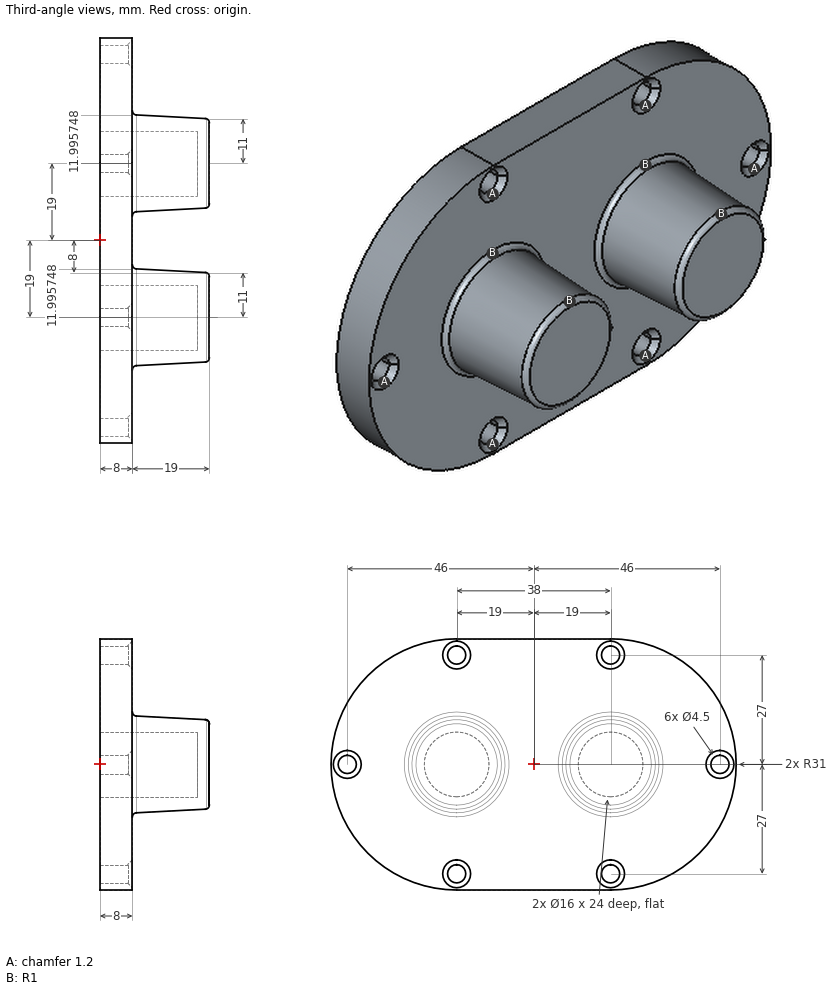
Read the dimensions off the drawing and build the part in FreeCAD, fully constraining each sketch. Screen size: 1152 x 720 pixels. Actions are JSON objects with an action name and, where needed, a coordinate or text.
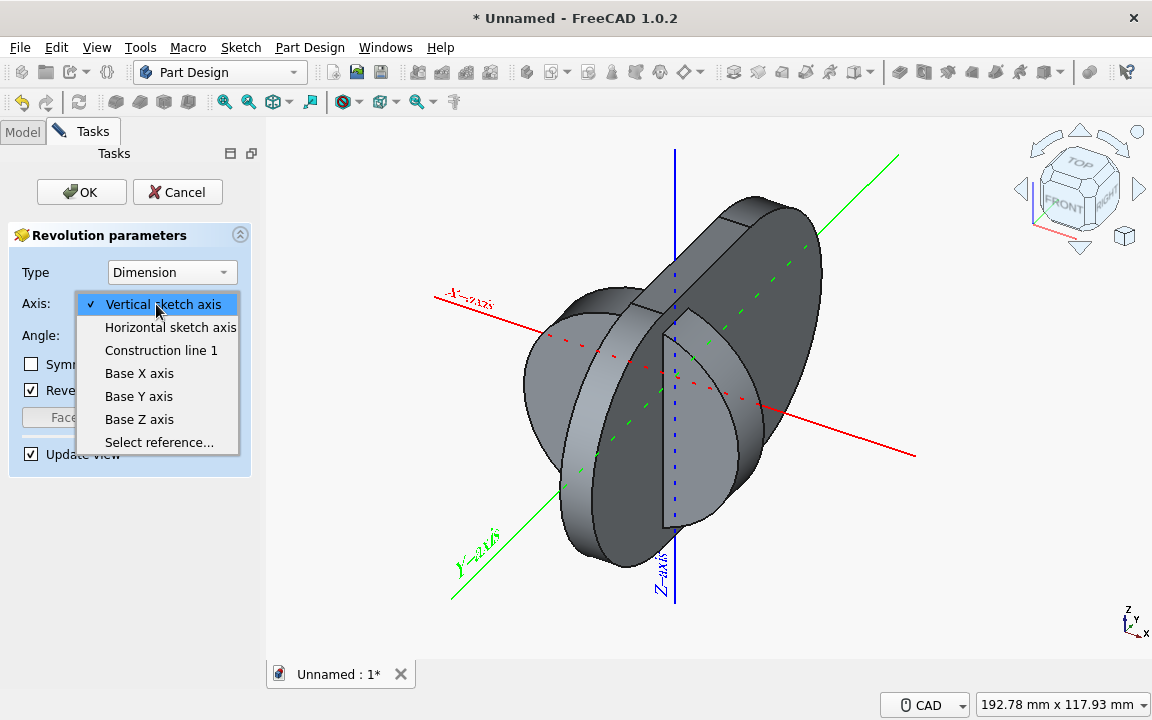
{"action": "left_click", "coordinate": [156, 350]}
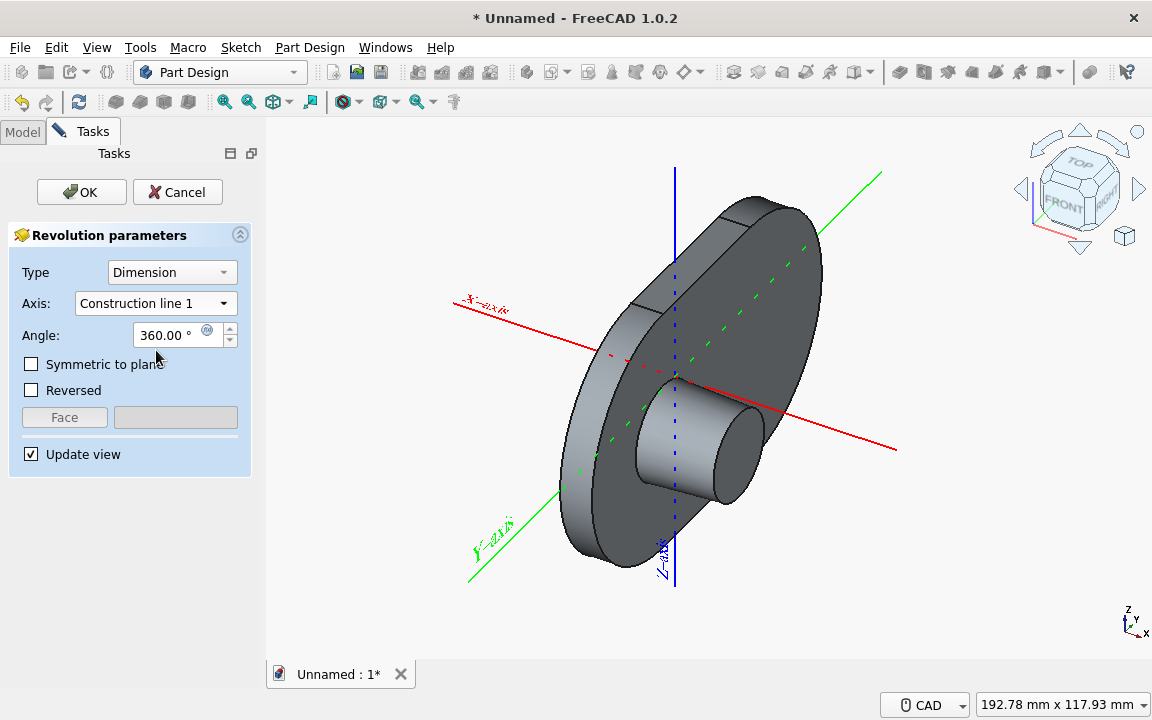
{"action": "left_click", "coordinate": [82, 192]}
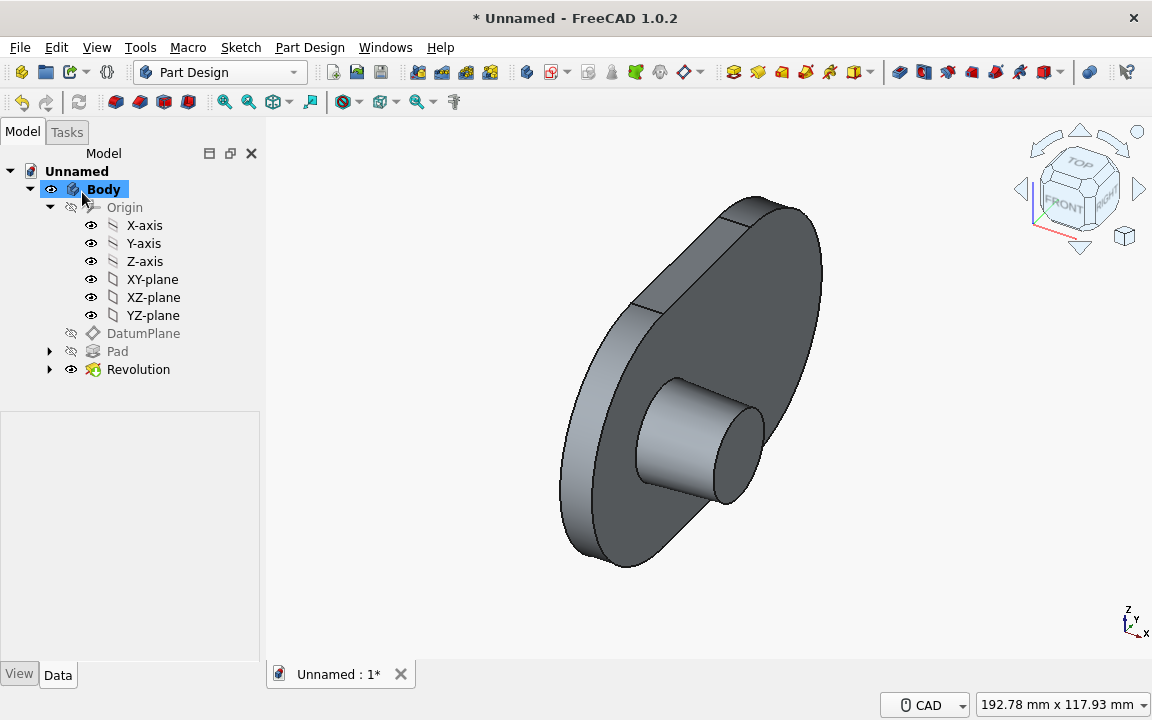
{"action": "left_click", "coordinate": [552, 72]}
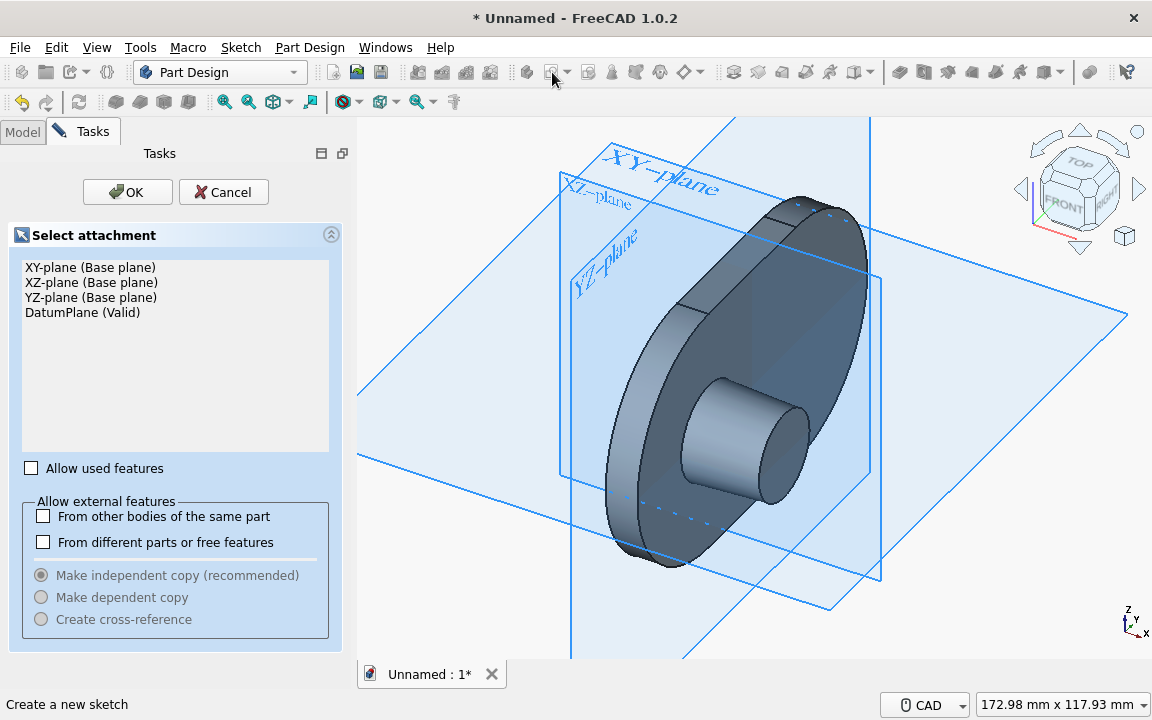
{"action": "left_click", "coordinate": [82, 268]}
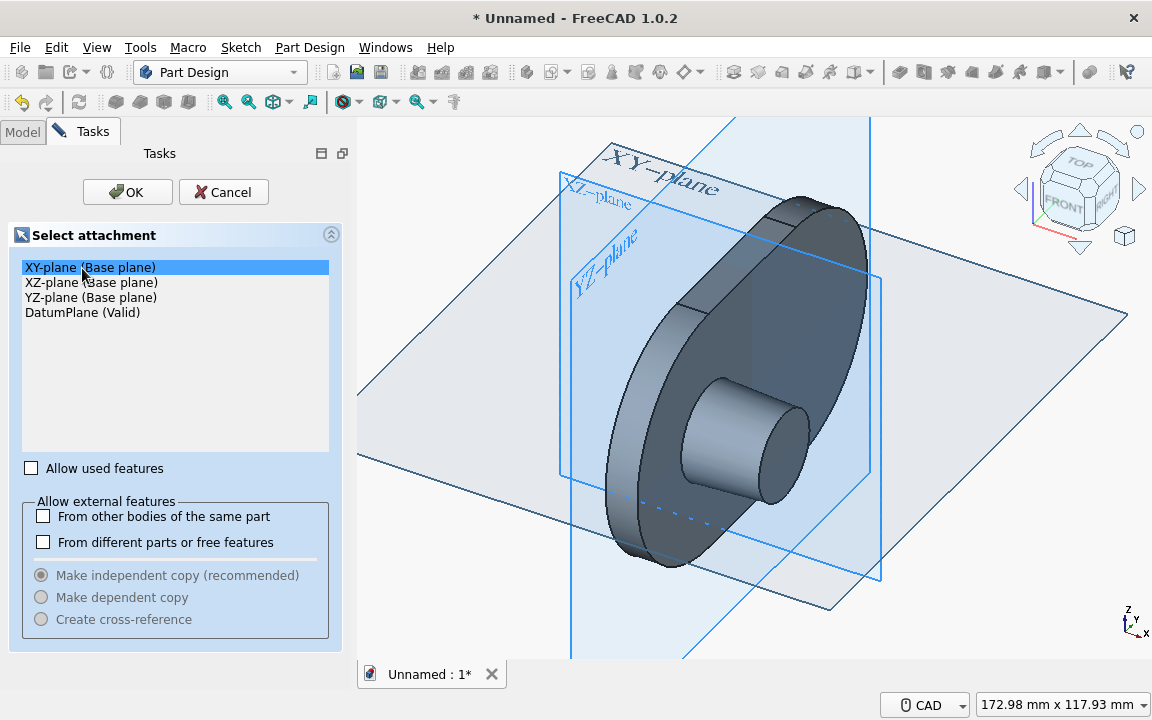
{"action": "left_click", "coordinate": [128, 192]}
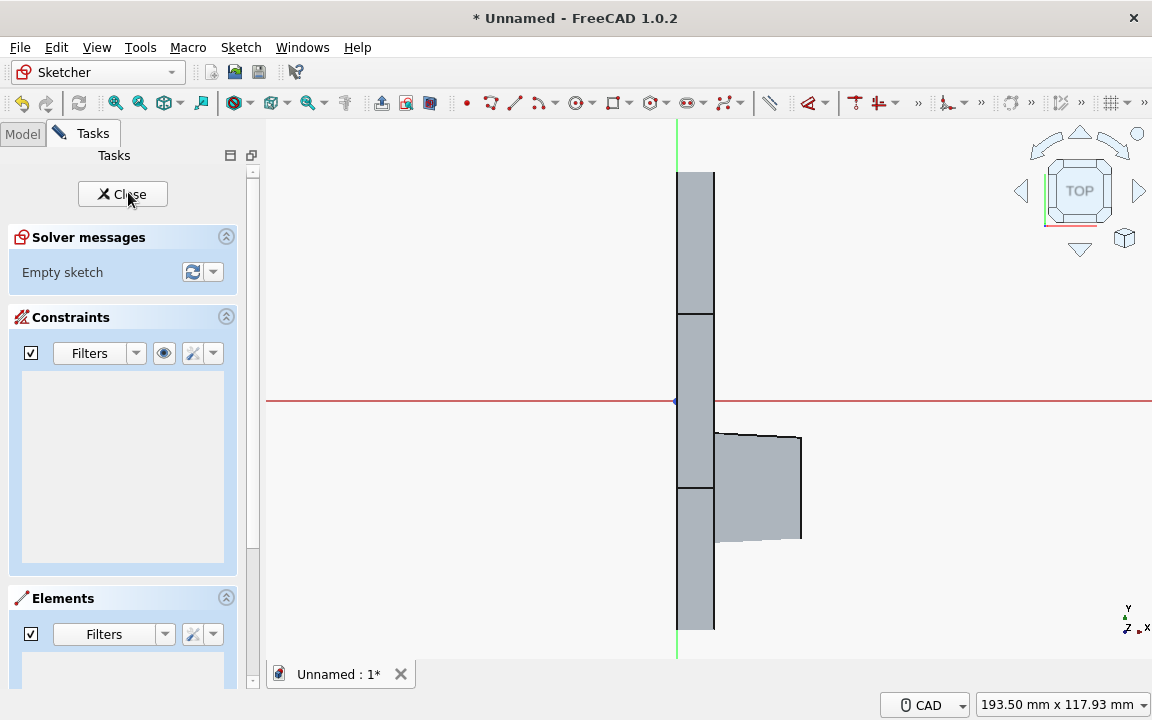
{"action": "left_click", "coordinate": [430, 104]}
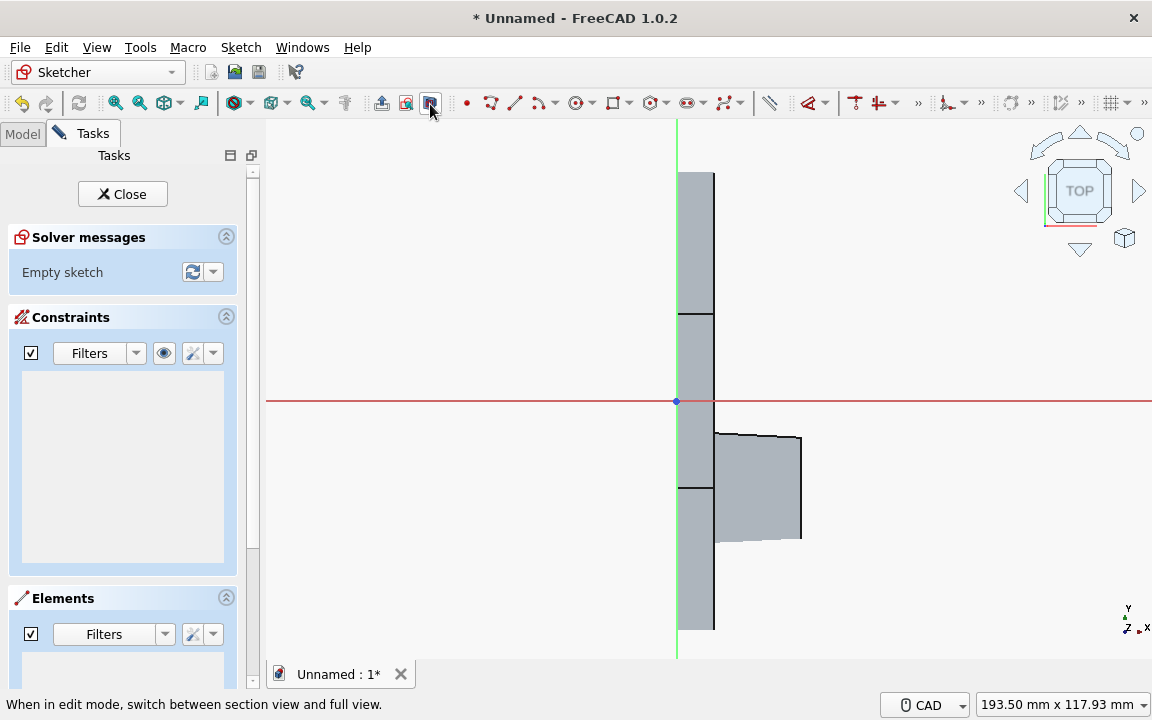
{"action": "scroll", "coordinate": [850, 282], "scroll_direction": "up", "scroll_amount": 4}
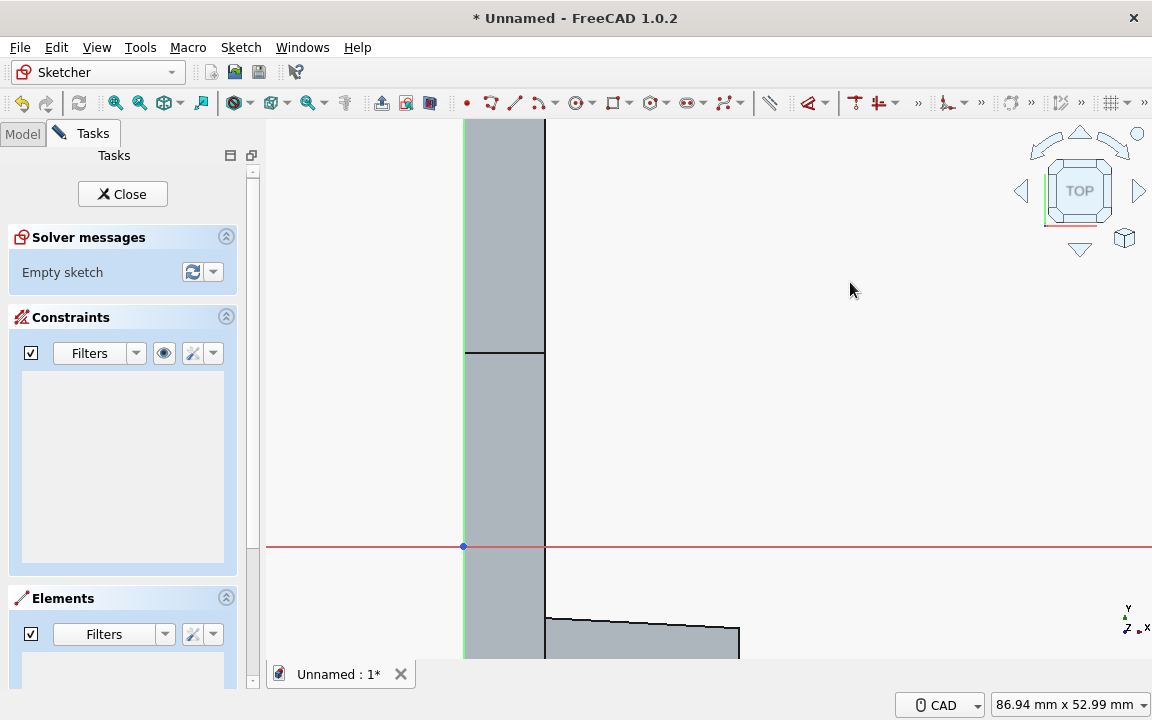
{"action": "left_click", "coordinate": [492, 104]}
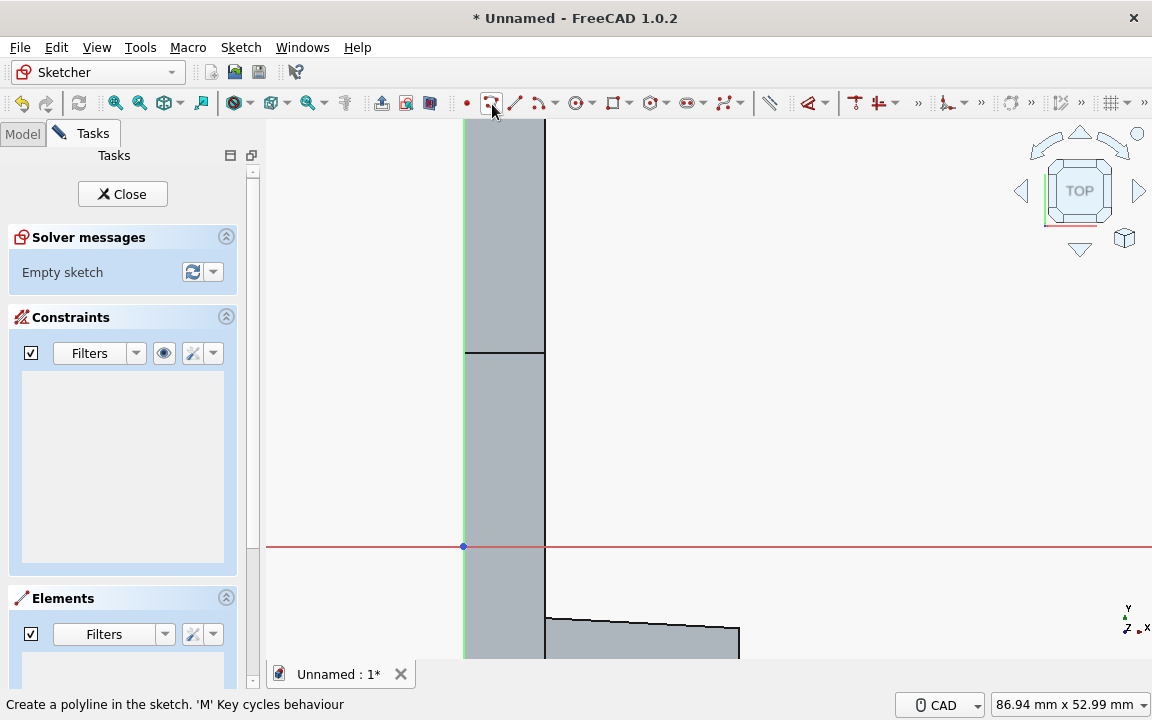
{"action": "left_click", "coordinate": [545, 353]}
{"action": "left_click", "coordinate": [739, 353]}
{"action": "left_click", "coordinate": [739, 241]}
{"action": "left_click", "coordinate": [545, 231]}
{"action": "left_click", "coordinate": [545, 354]}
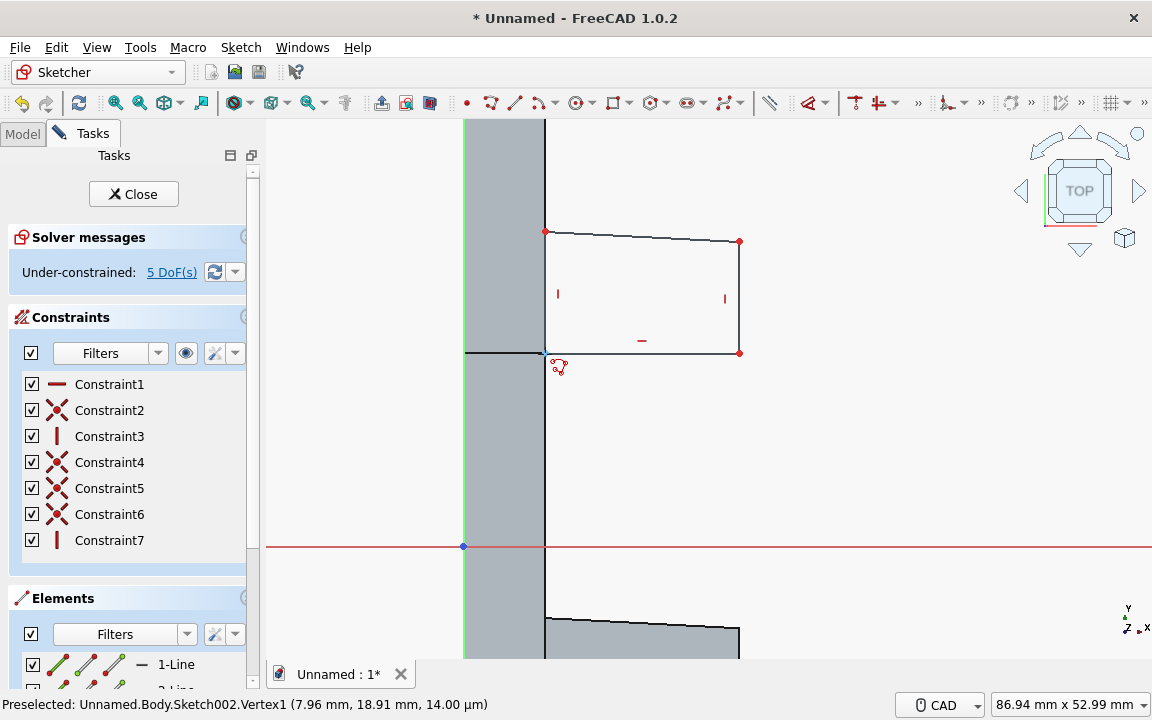
{"action": "left_click", "coordinate": [516, 104]}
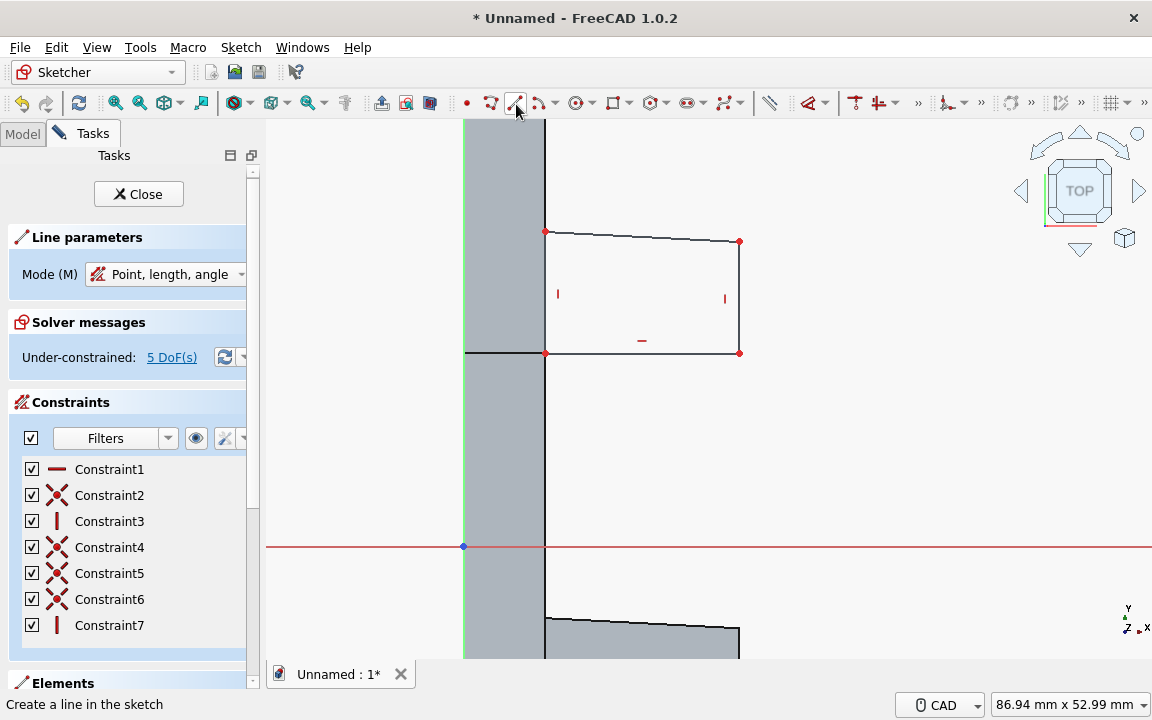
{"action": "left_click", "coordinate": [758, 353]}
{"action": "left_click", "coordinate": [817, 353]}
{"action": "key", "text": "Escape"}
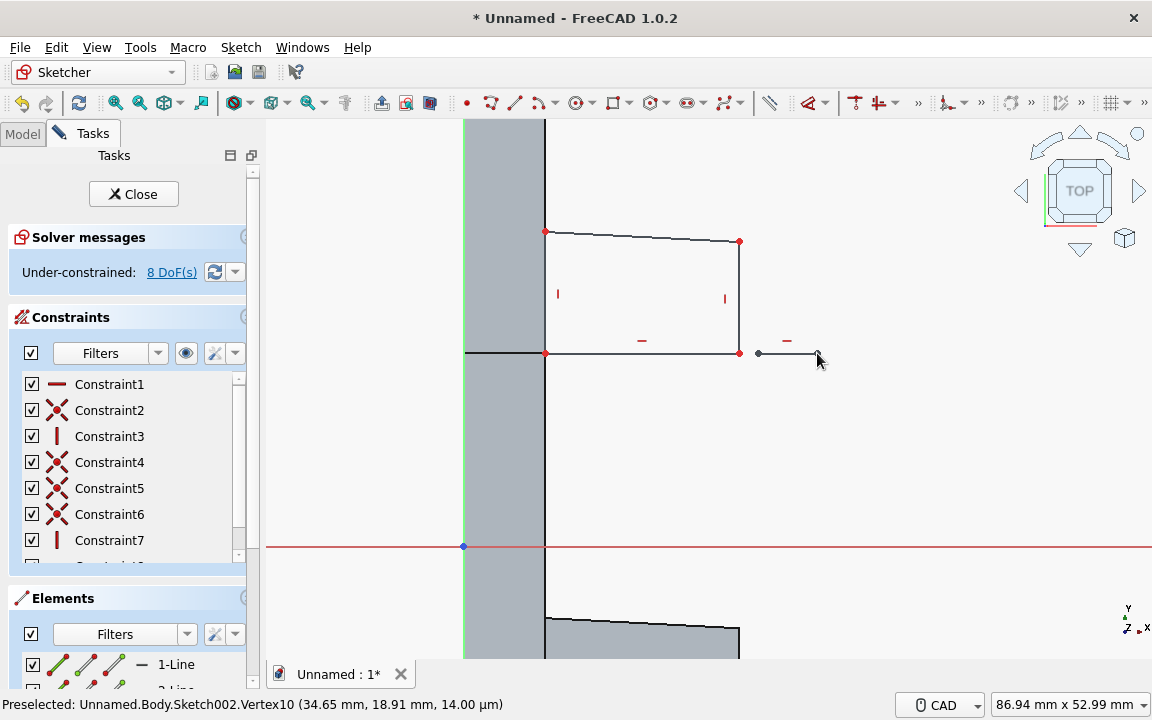
{"action": "left_click", "coordinate": [776, 354]}